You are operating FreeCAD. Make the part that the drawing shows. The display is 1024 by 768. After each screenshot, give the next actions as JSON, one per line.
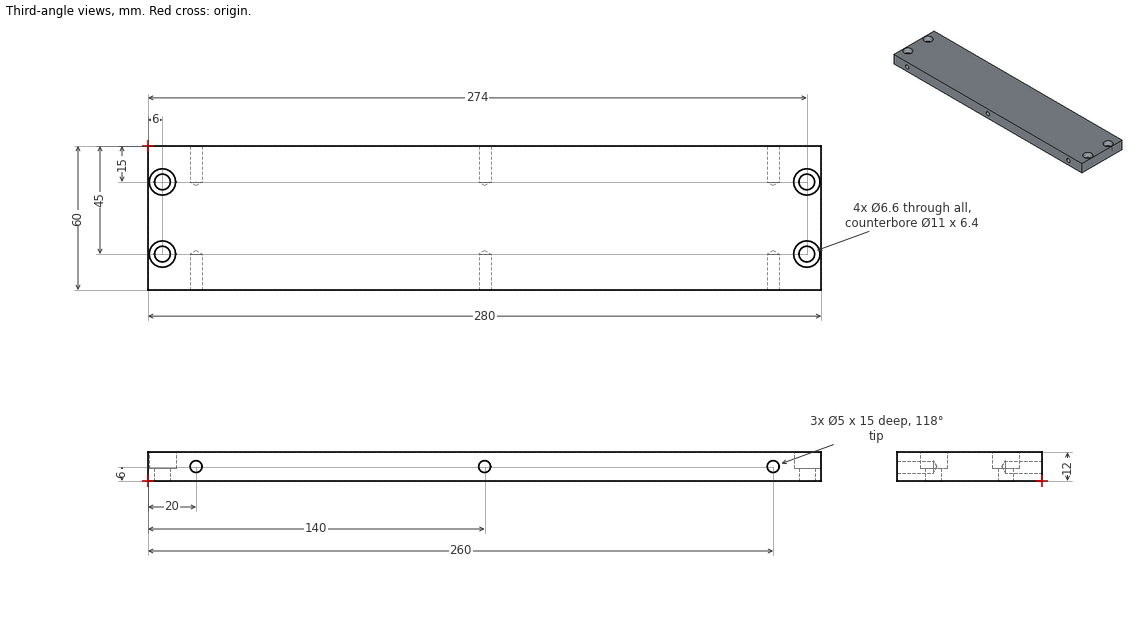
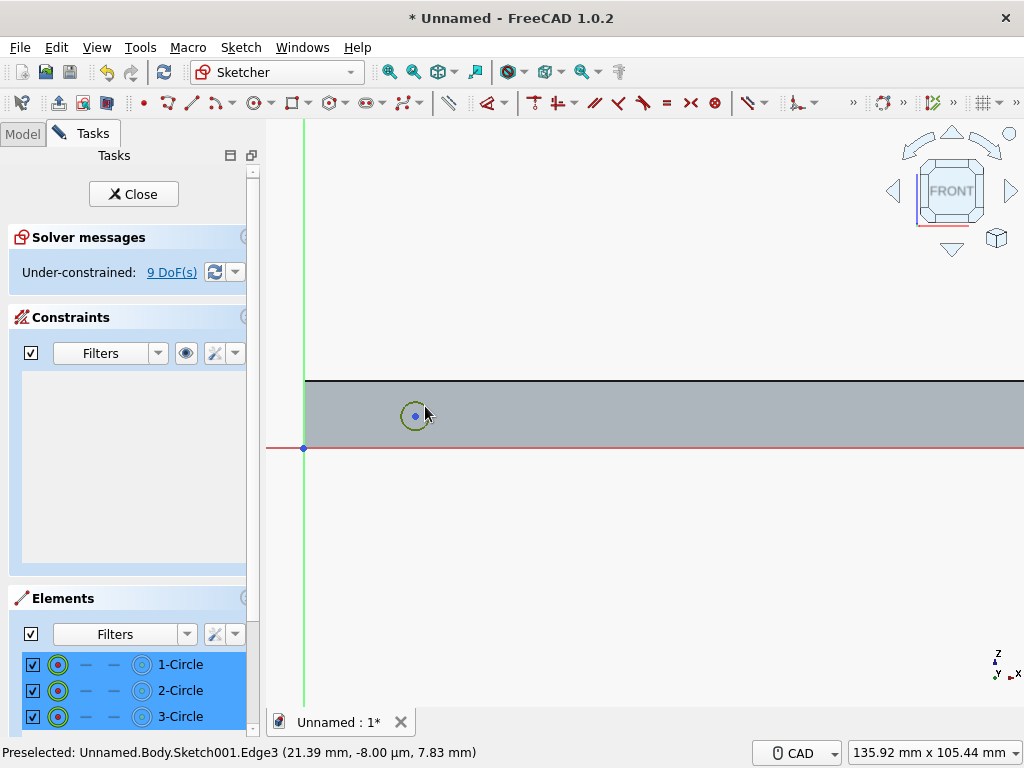
{"action": "left_click", "coordinate": [668, 104]}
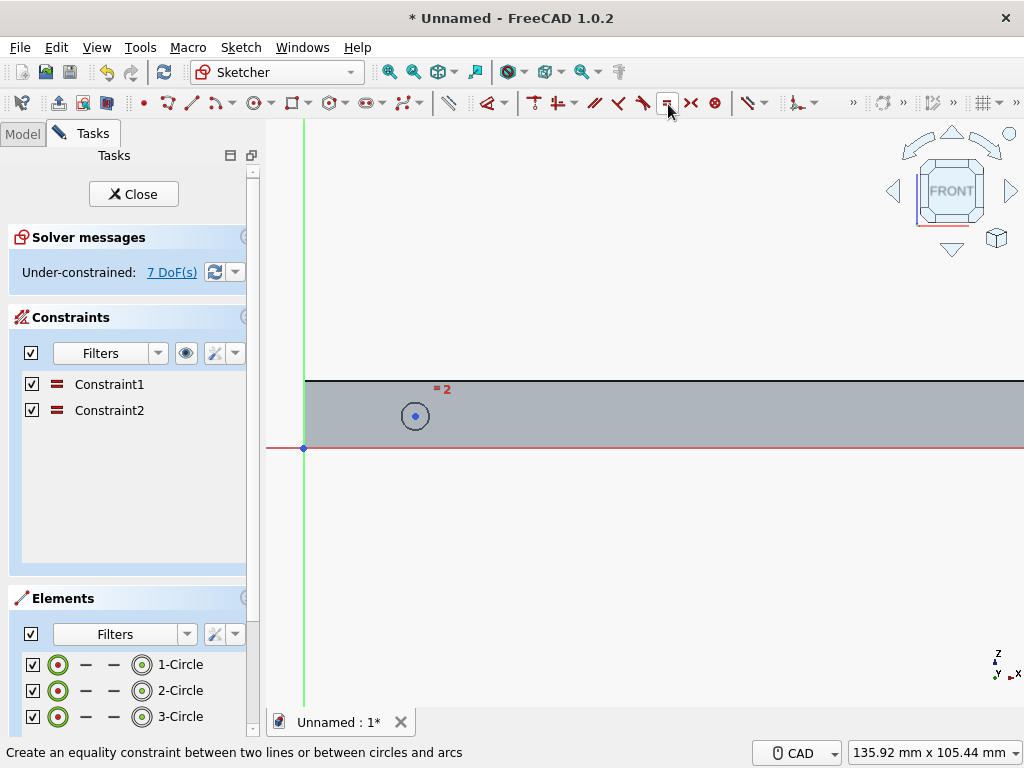
{"action": "left_click", "coordinate": [488, 104]}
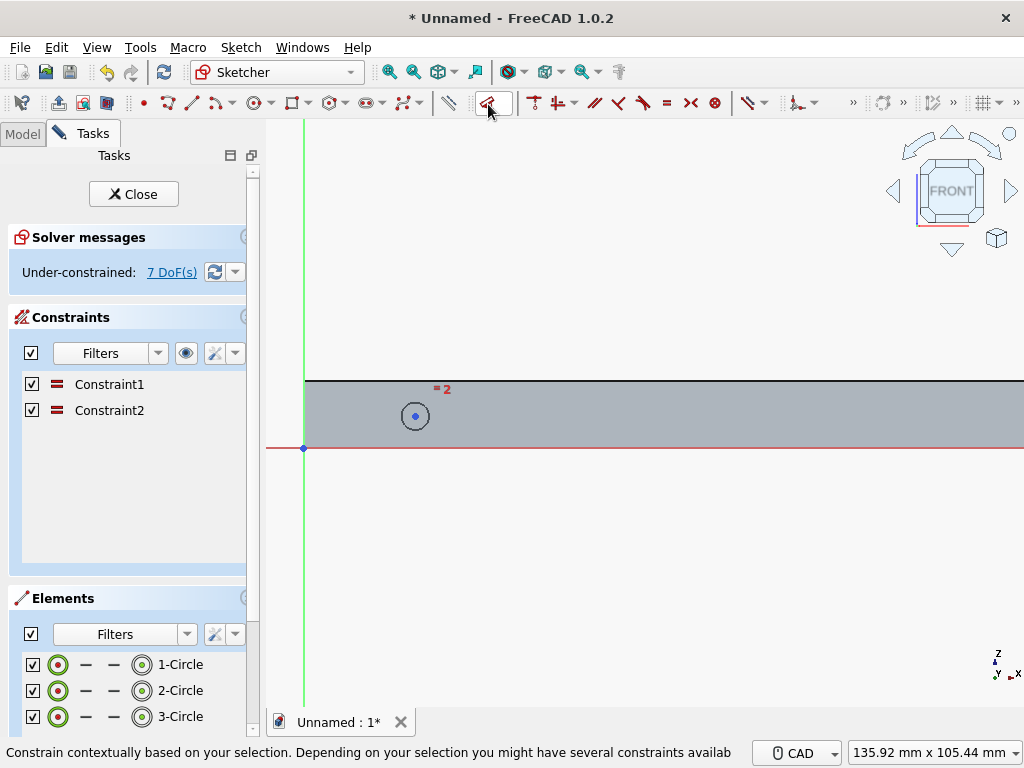
{"action": "scroll", "coordinate": [426, 409], "scroll_direction": "down", "scroll_amount": 7}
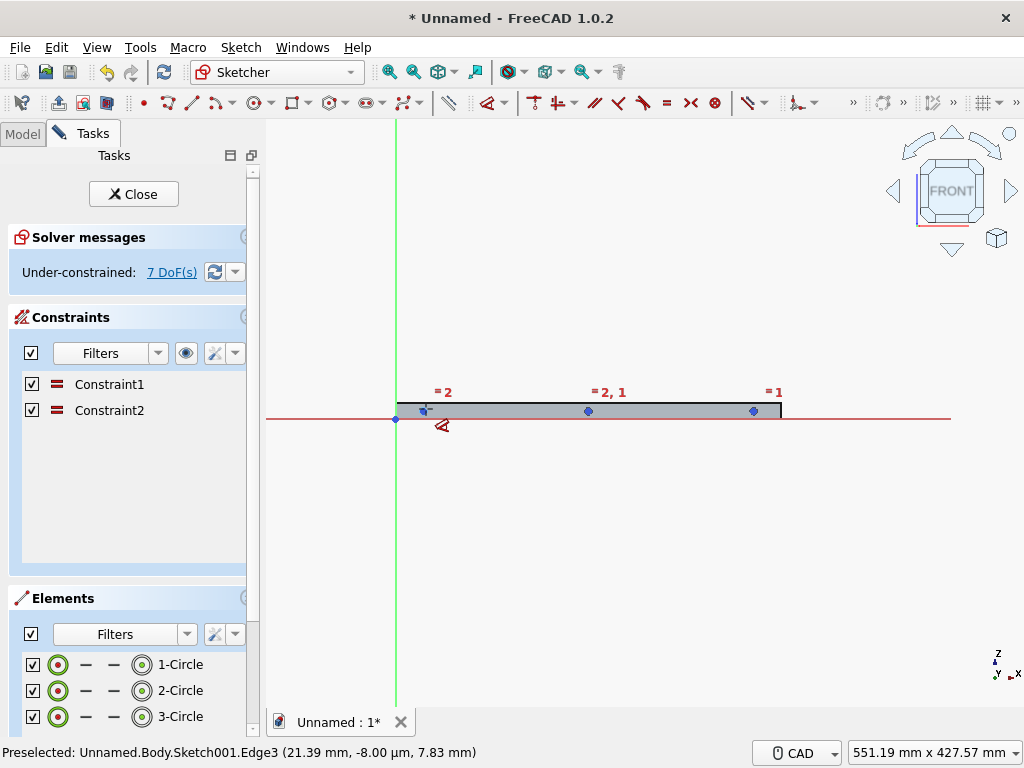
{"action": "scroll", "coordinate": [756, 409], "scroll_direction": "up", "scroll_amount": 9}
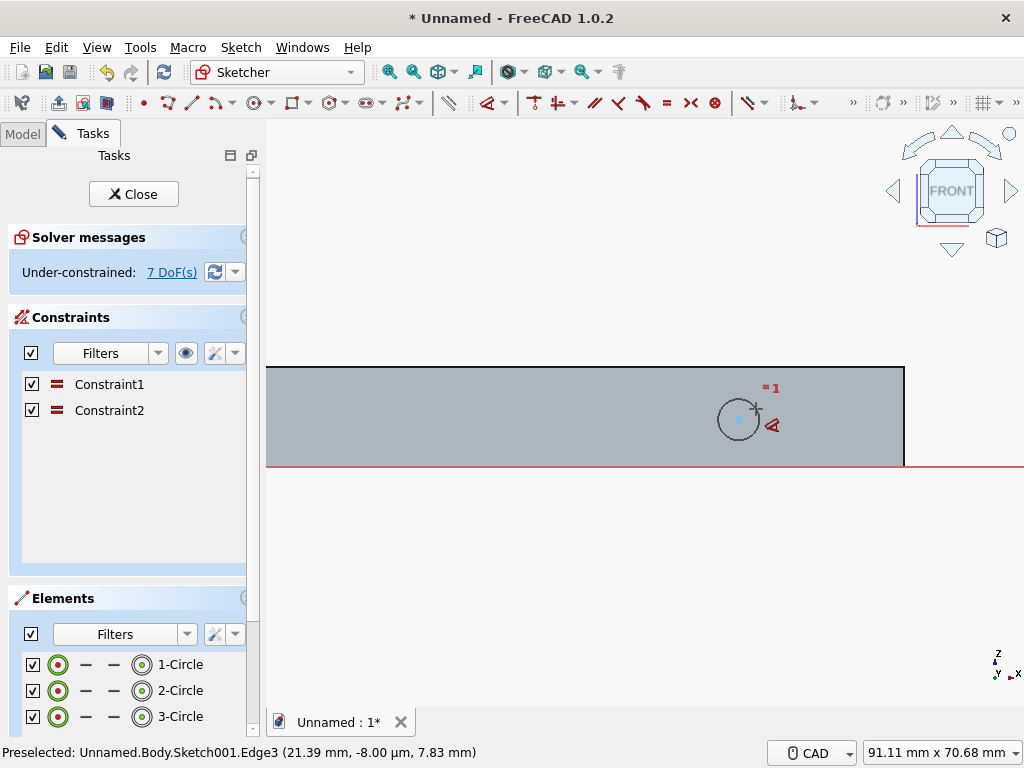
{"action": "left_click", "coordinate": [753, 405]}
{"action": "left_click", "coordinate": [775, 382]}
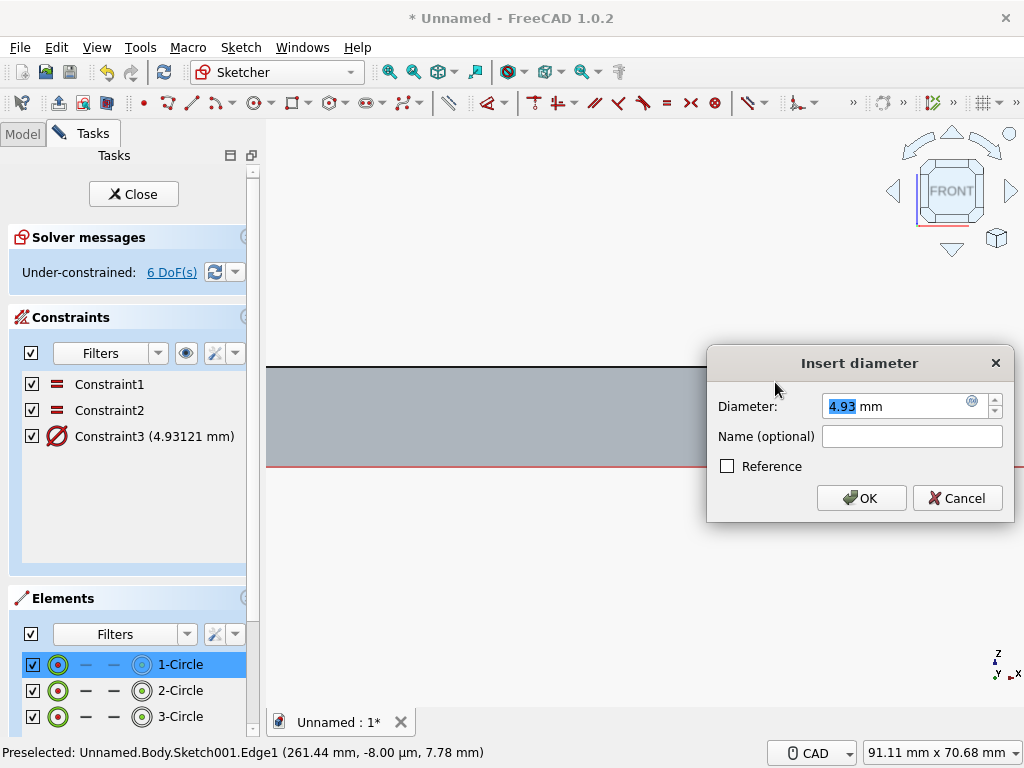
{"action": "type", "text": "5"}
{"action": "key", "text": "Return"}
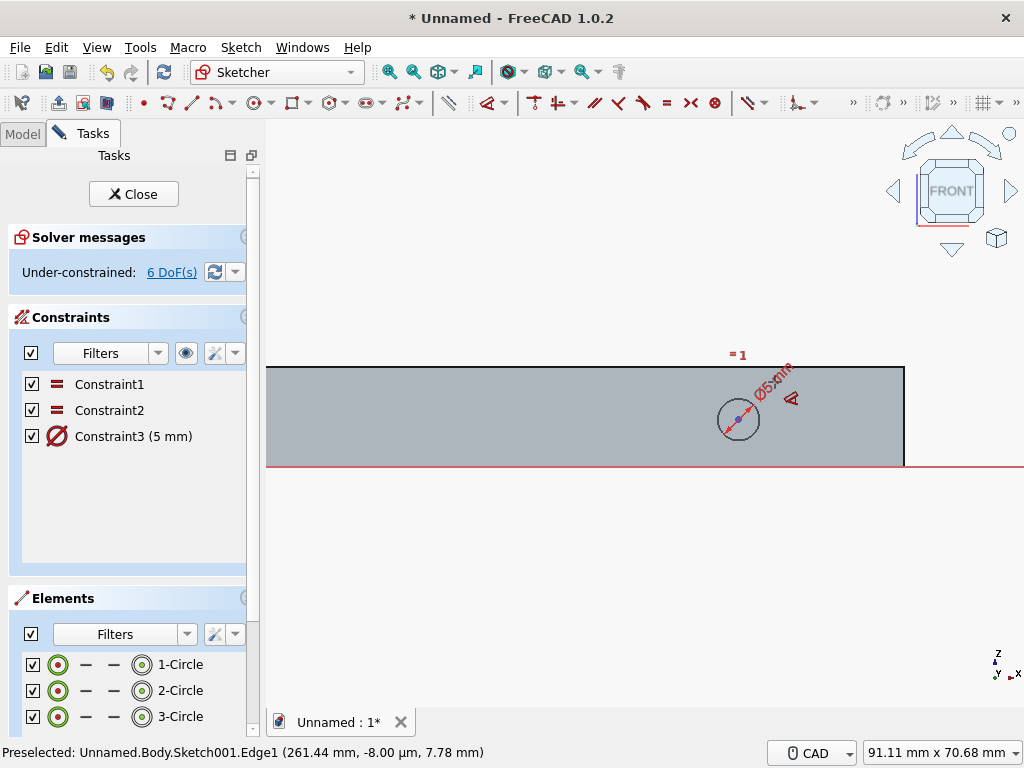
{"action": "left_click", "coordinate": [739, 420]}
{"action": "left_click", "coordinate": [773, 443]}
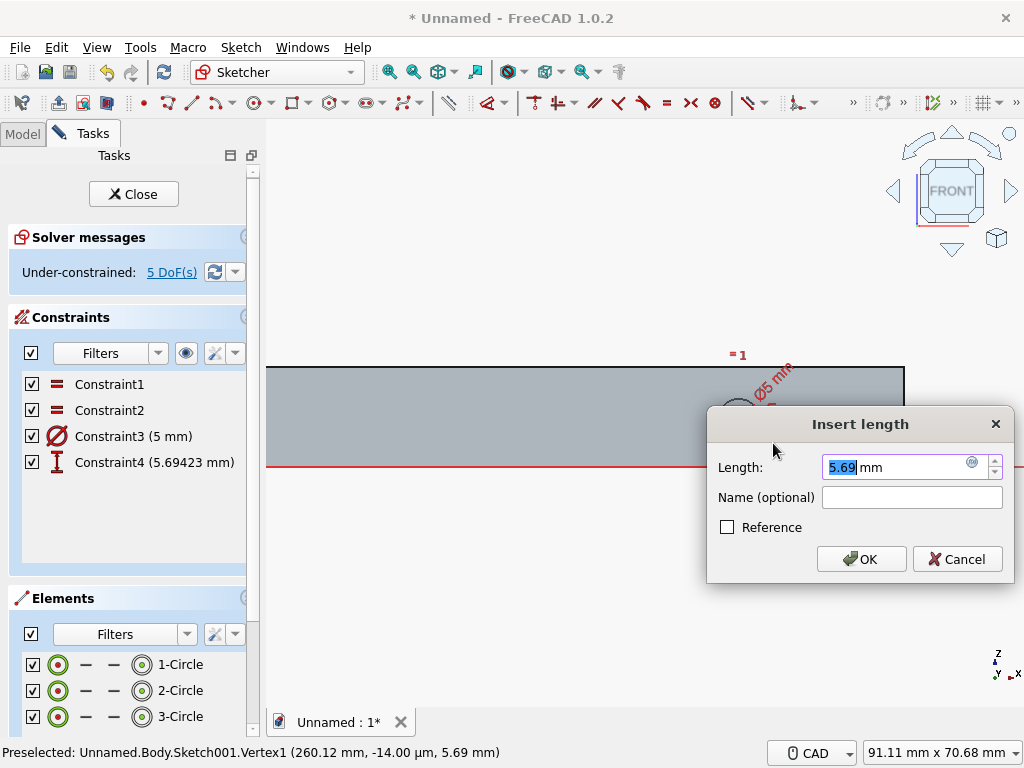
{"action": "type", "text": "6"}
{"action": "key", "text": "Return"}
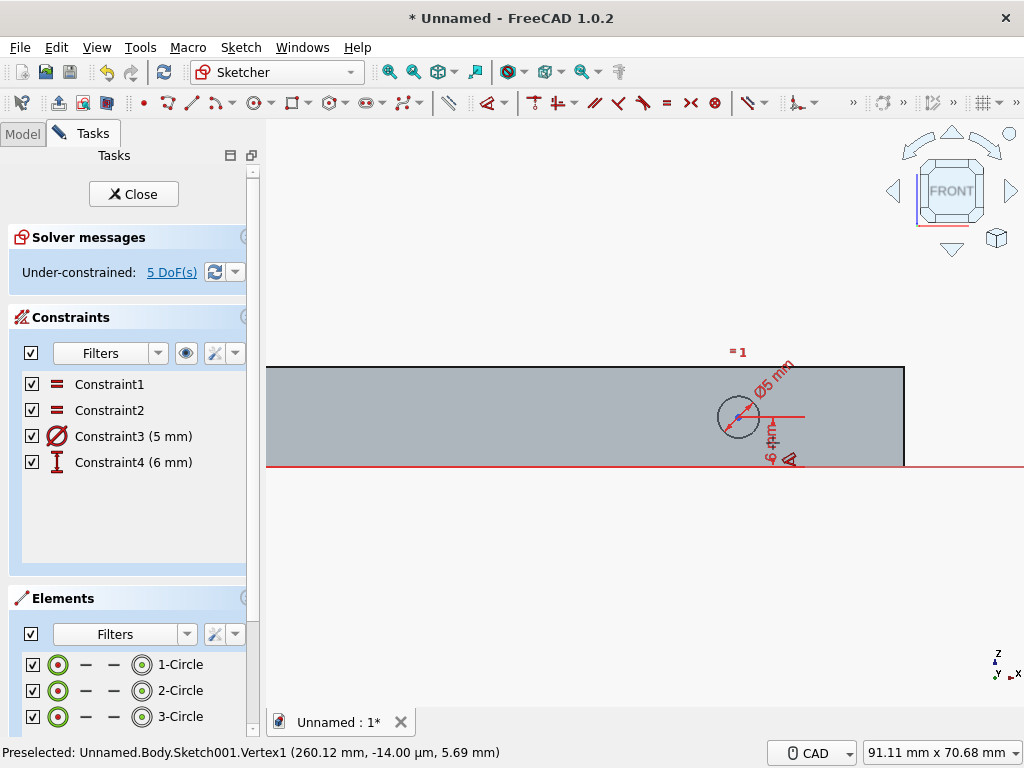
{"action": "scroll", "coordinate": [757, 409], "scroll_direction": "down", "scroll_amount": 9}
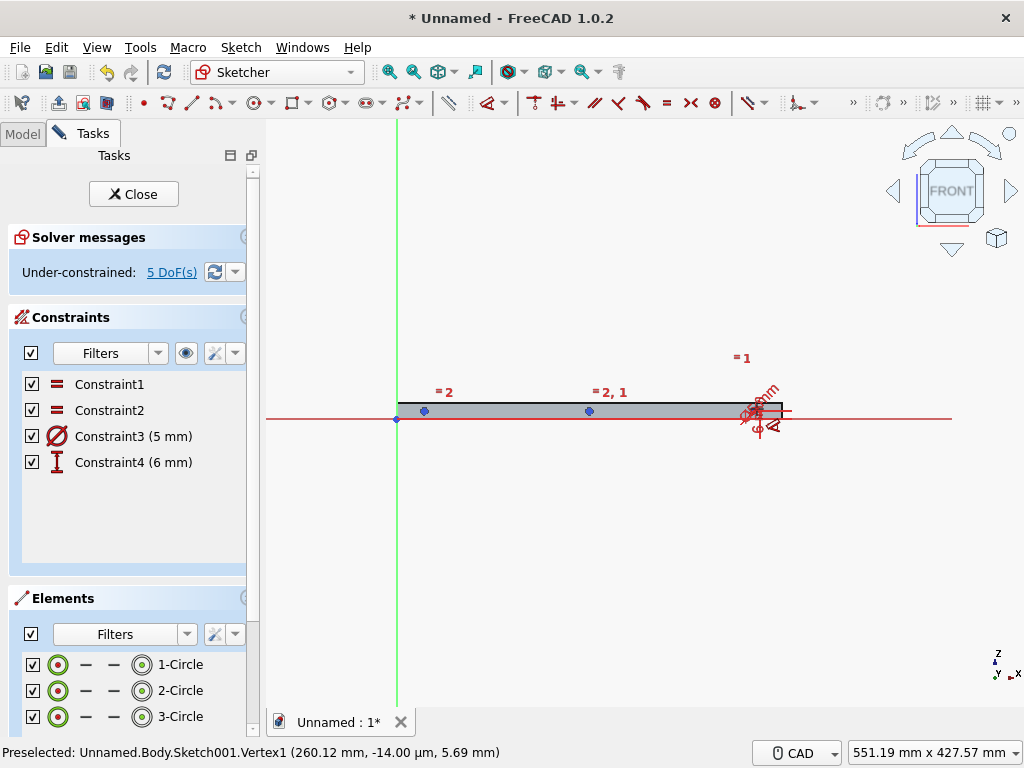
{"action": "scroll", "coordinate": [589, 411], "scroll_direction": "up", "scroll_amount": 8}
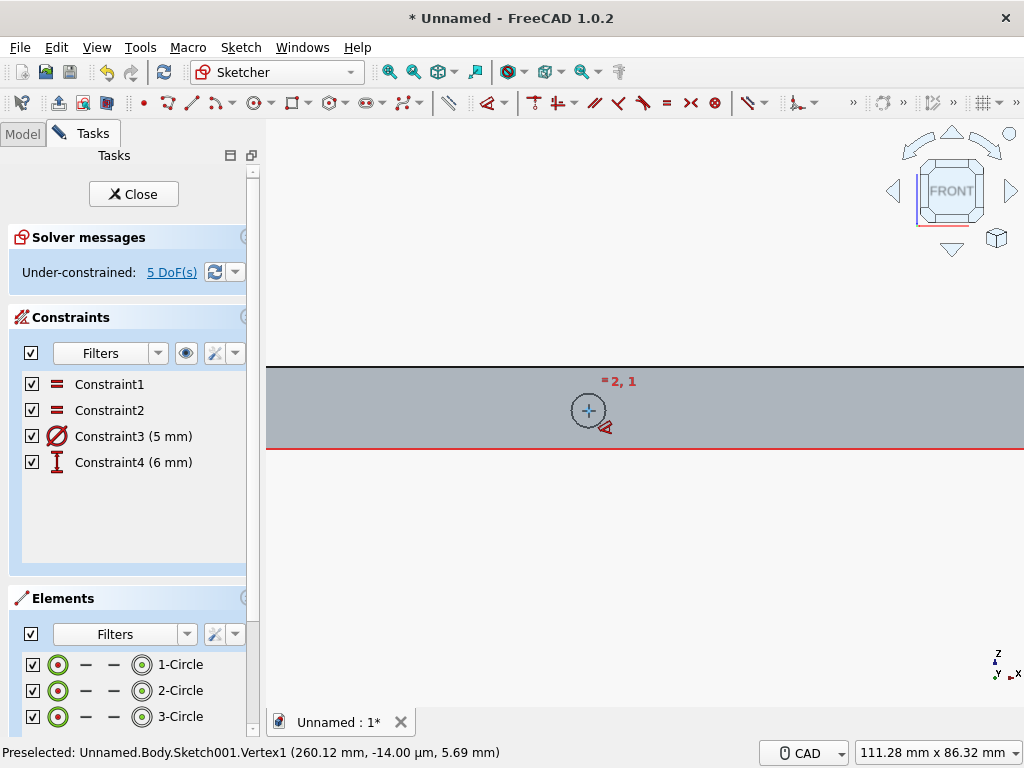
{"action": "left_click", "coordinate": [588, 411]}
{"action": "left_click", "coordinate": [622, 430]}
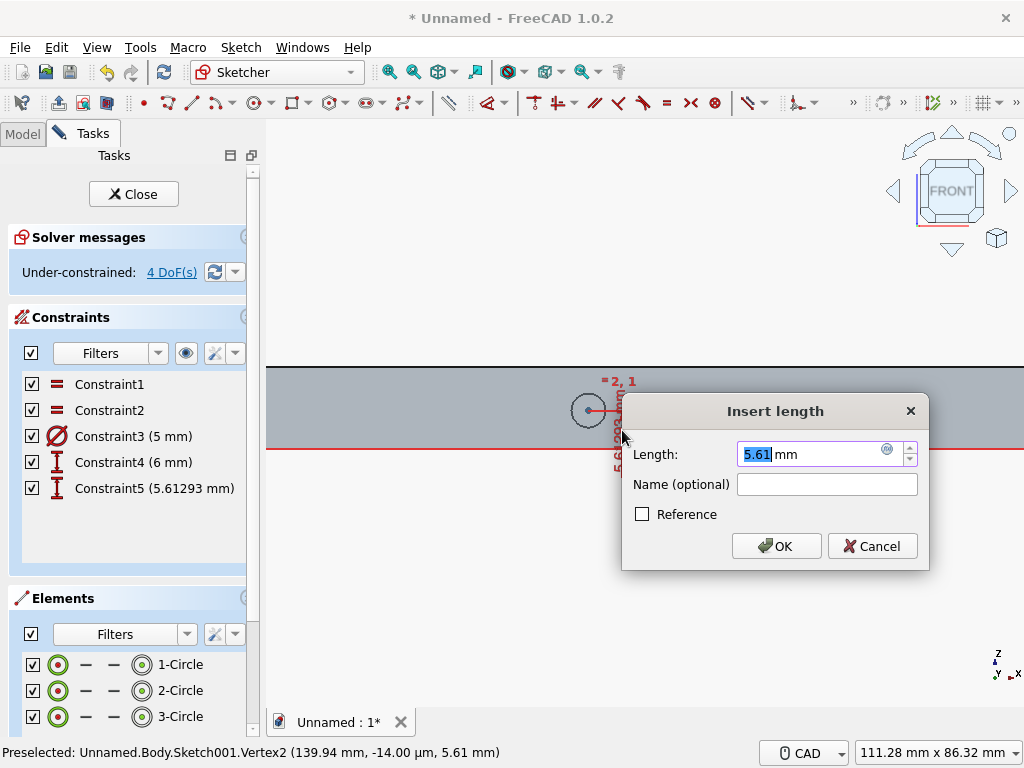
{"action": "type", "text": "6"}
{"action": "key", "text": "Return"}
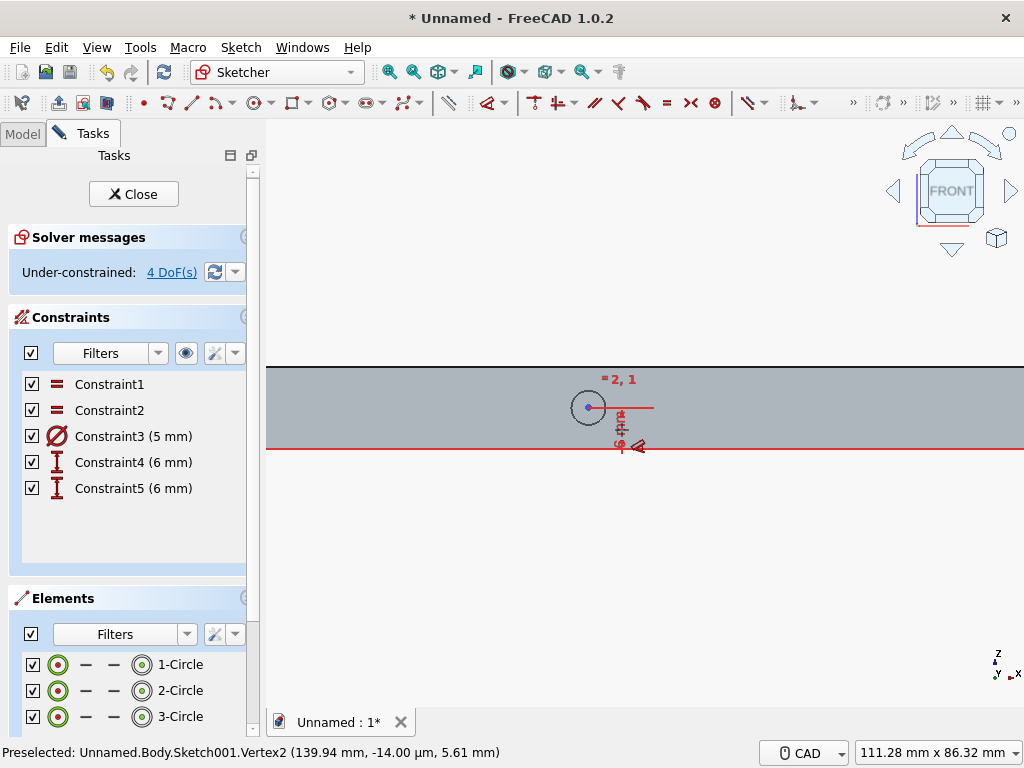
{"action": "scroll", "coordinate": [588, 411], "scroll_direction": "down", "scroll_amount": 8}